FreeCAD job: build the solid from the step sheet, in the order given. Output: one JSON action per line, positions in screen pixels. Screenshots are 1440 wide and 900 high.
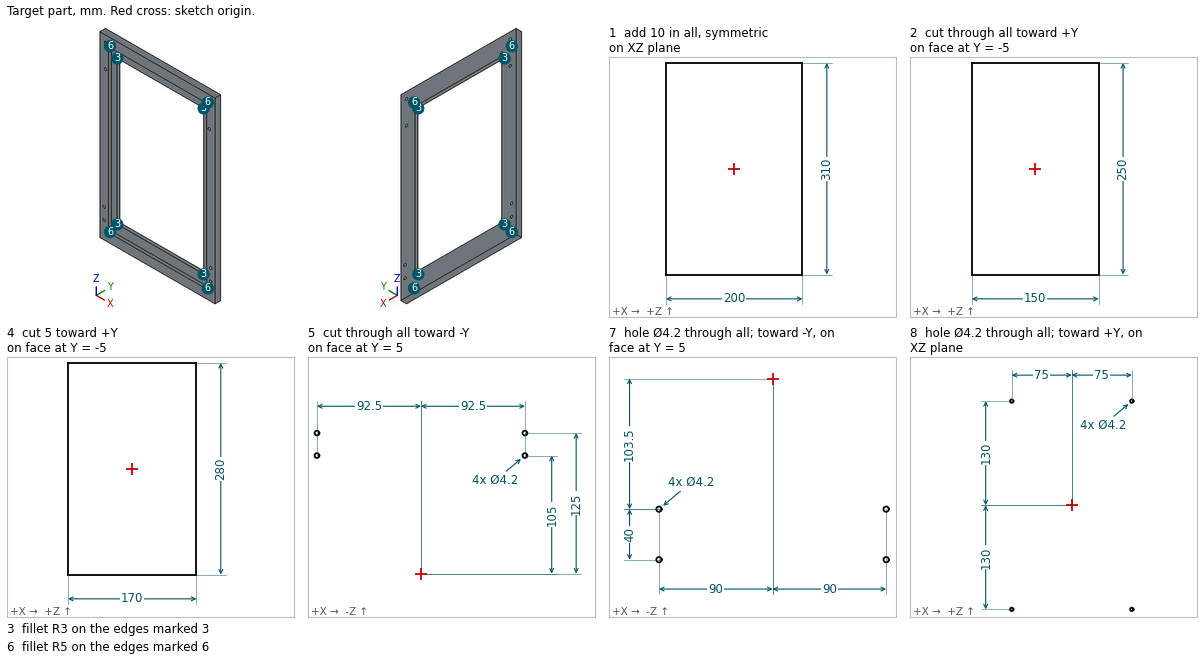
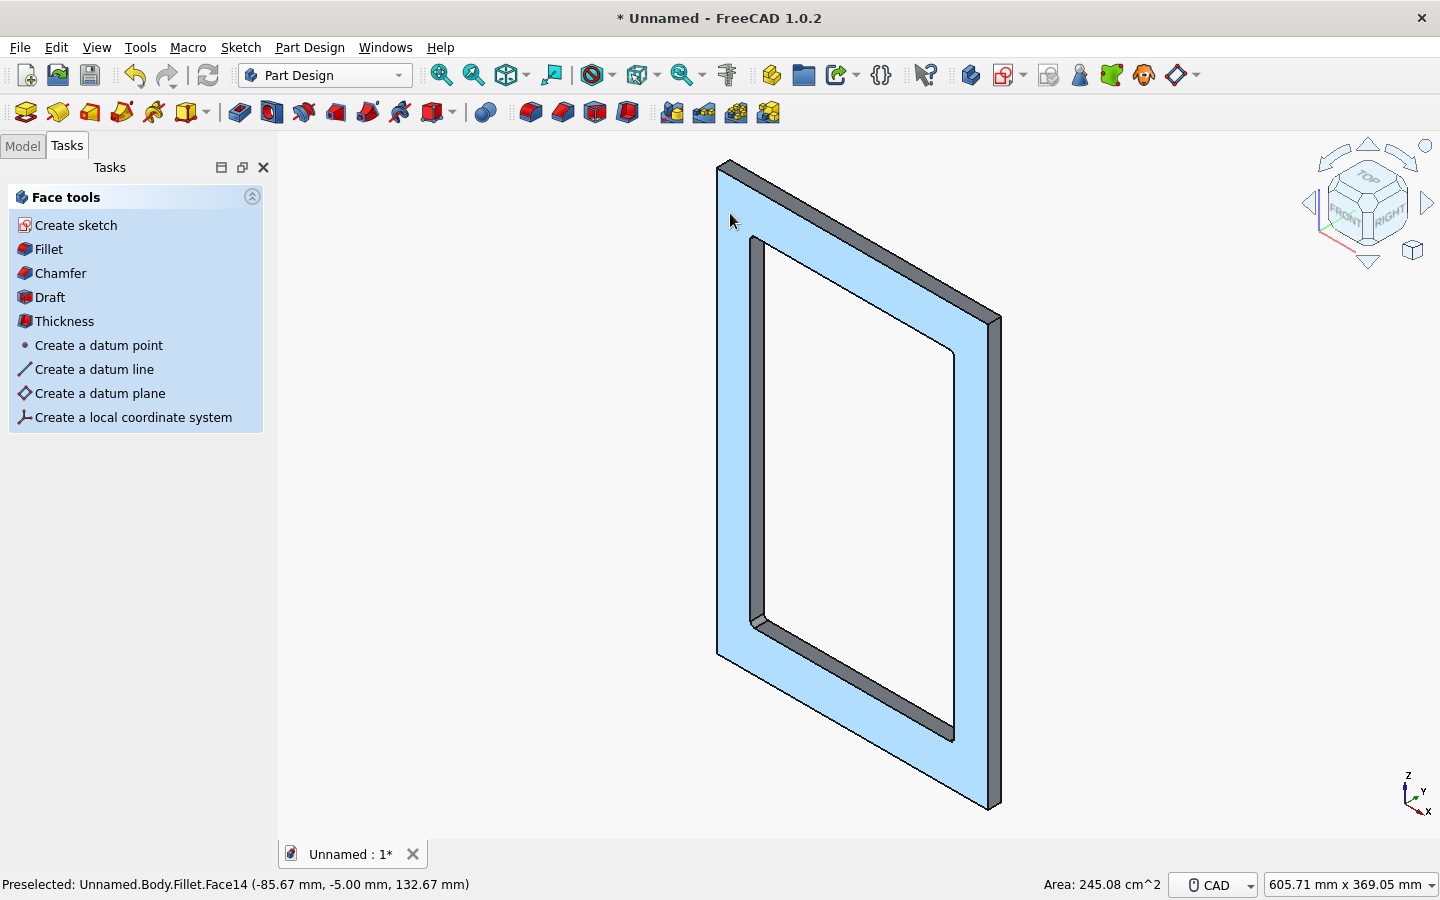
{"action": "left_click", "coordinate": [1004, 76]}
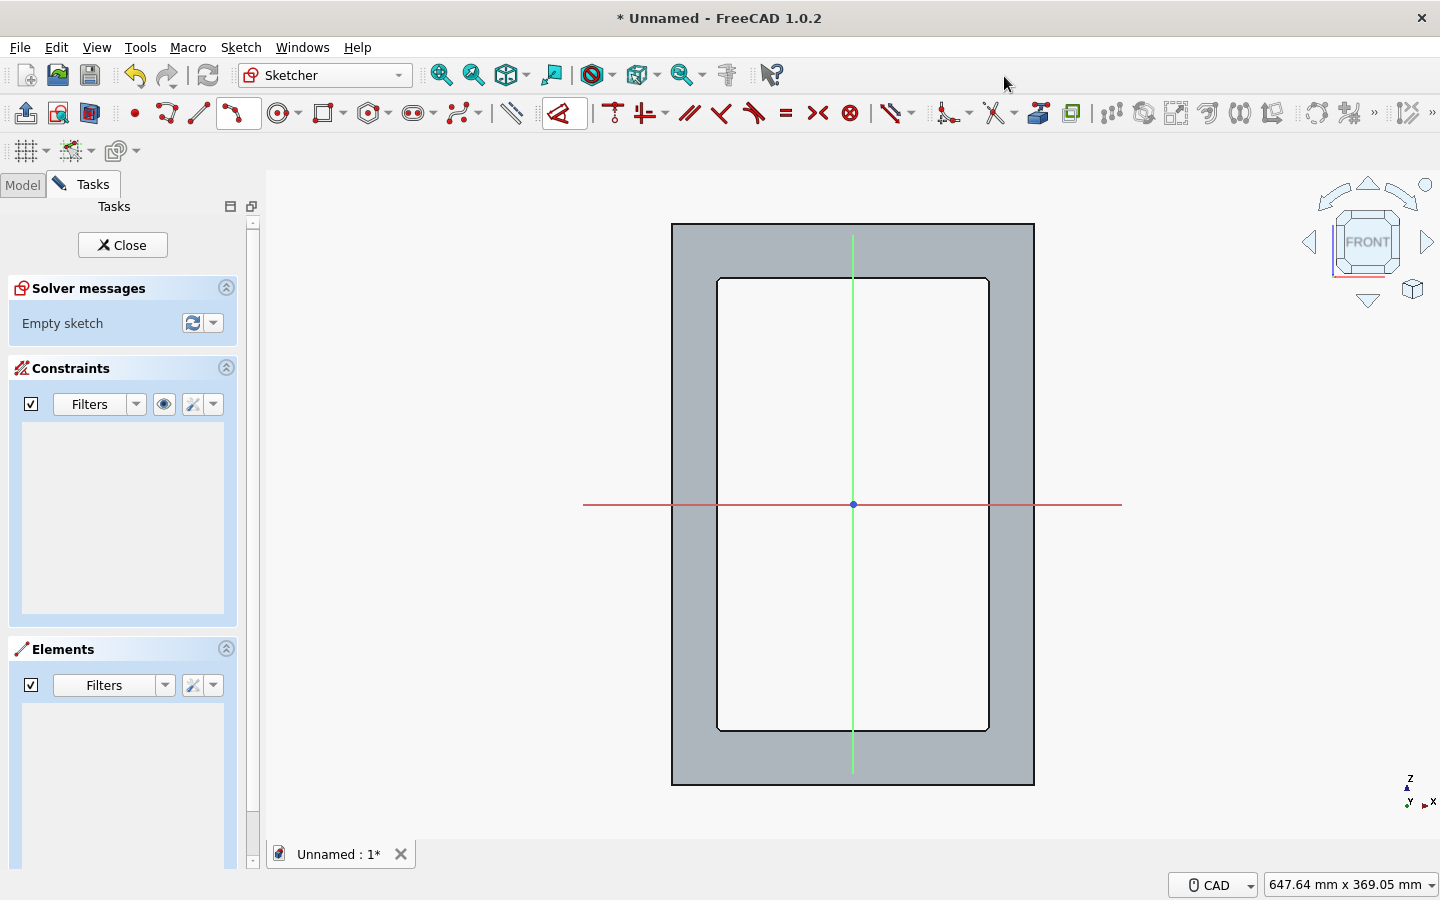
{"action": "key", "text": "g v"}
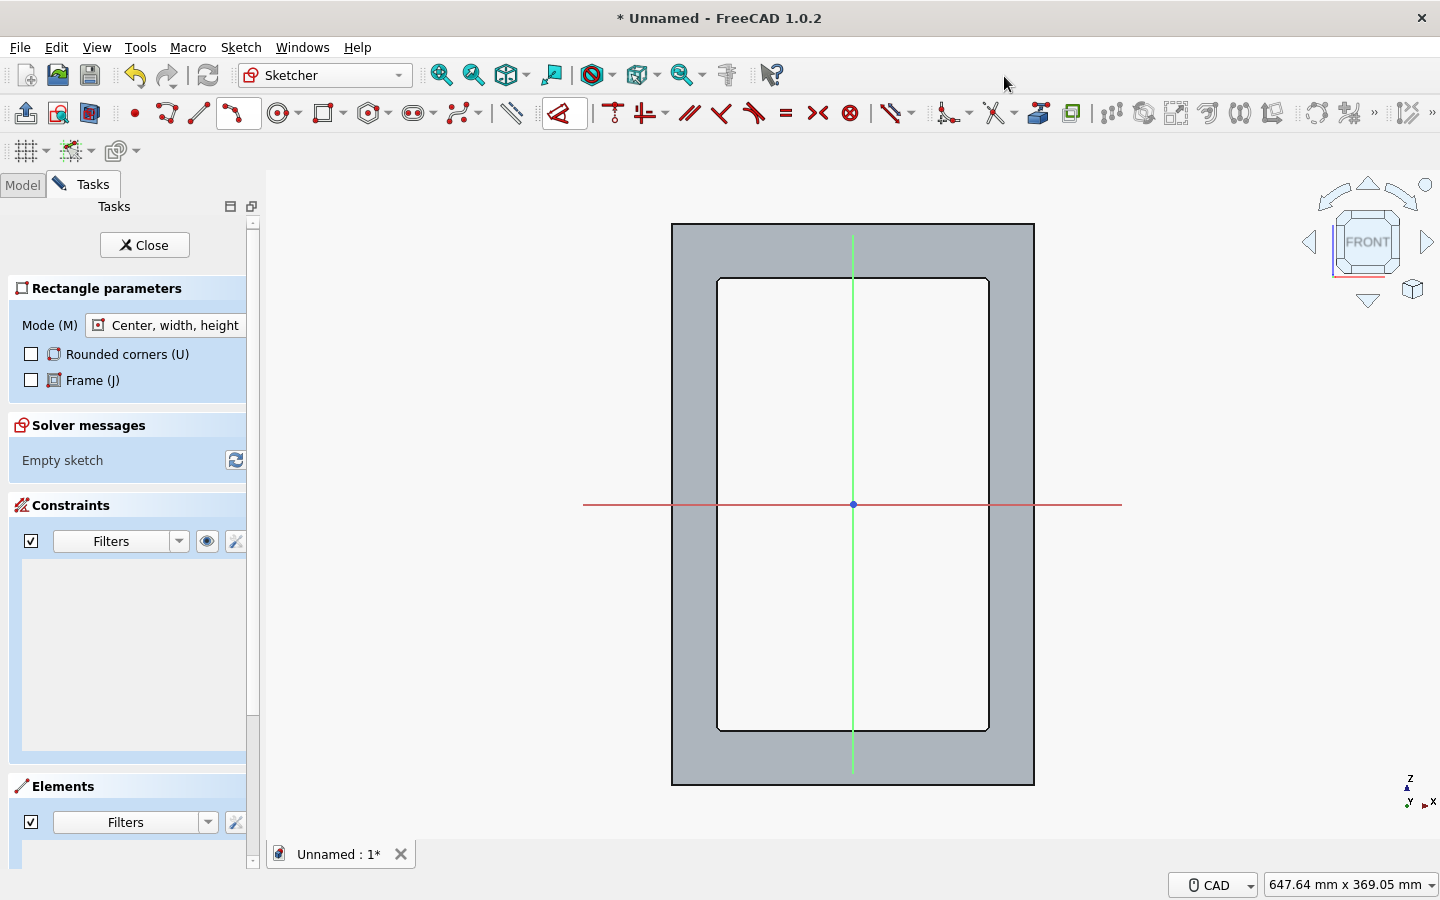
{"action": "left_click", "coordinate": [853, 504]}
{"action": "left_click", "coordinate": [1007, 251]}
{"action": "key", "text": "Escape"}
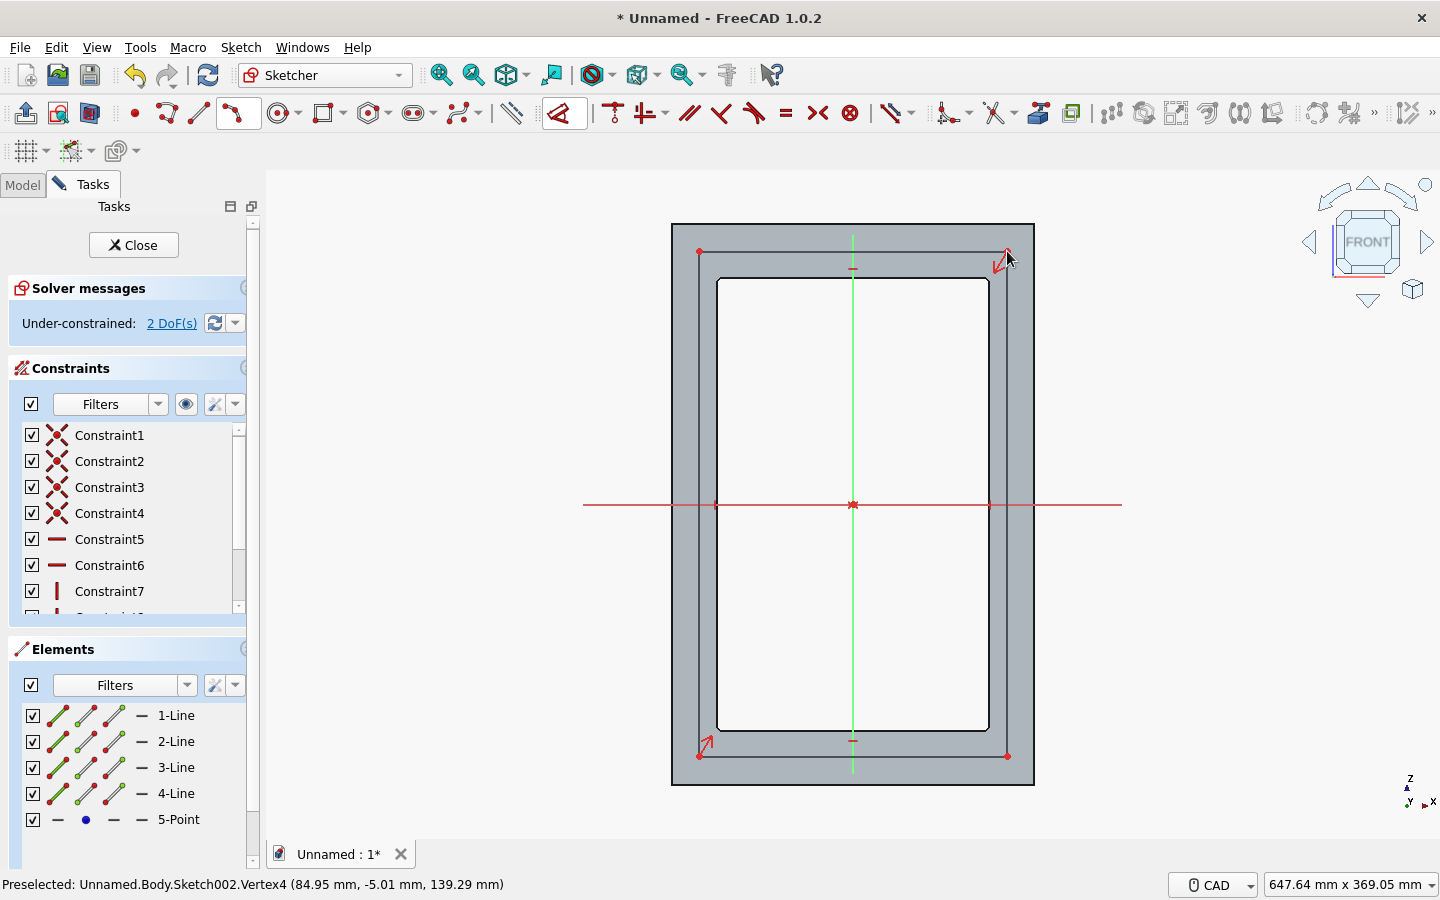
{"action": "left_click", "coordinate": [791, 757]}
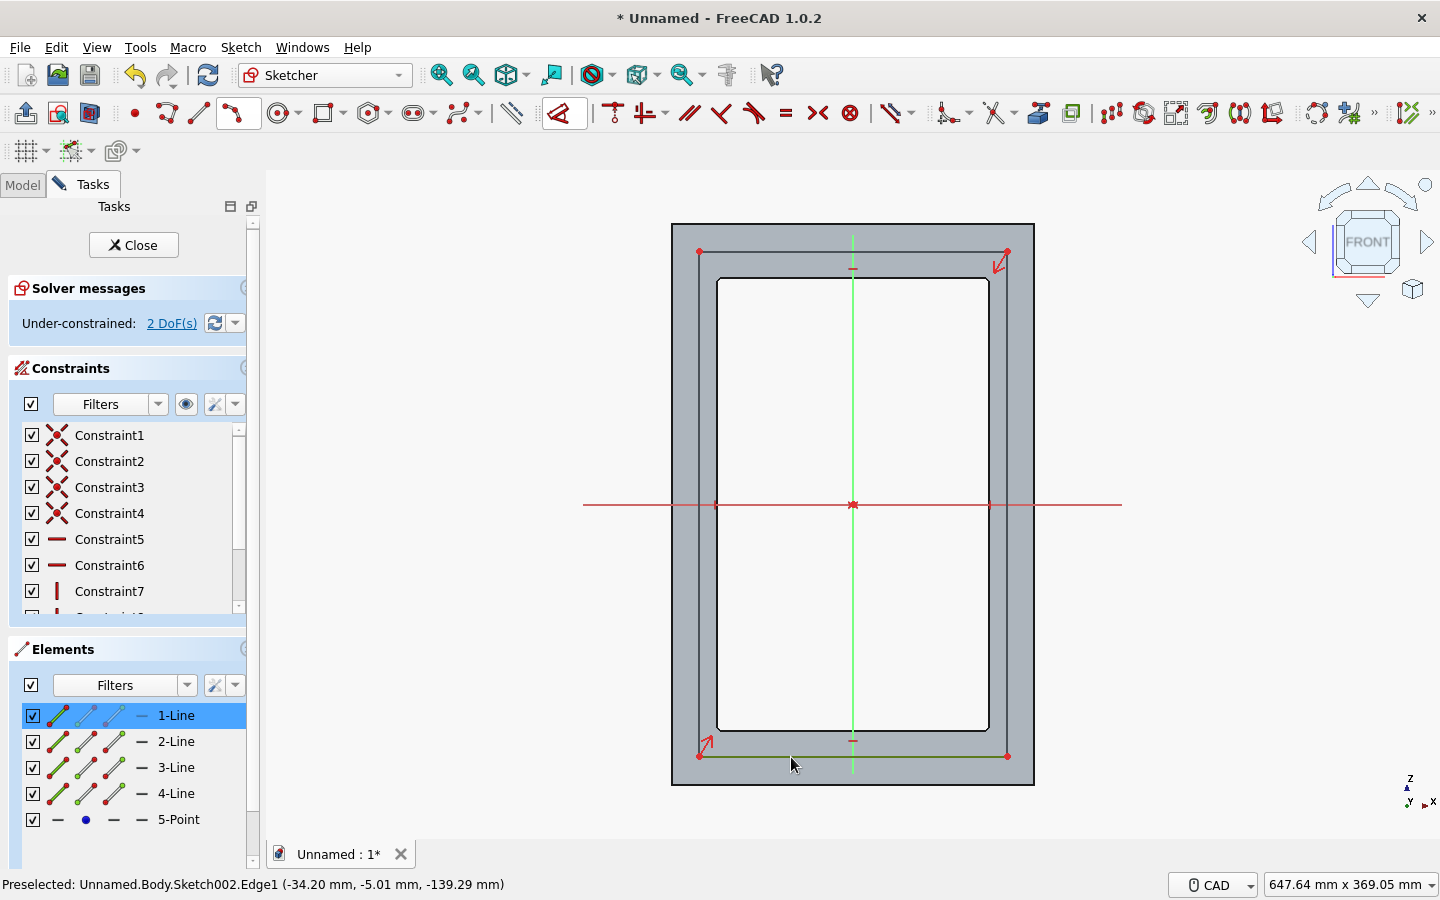
{"action": "key", "text": "l"}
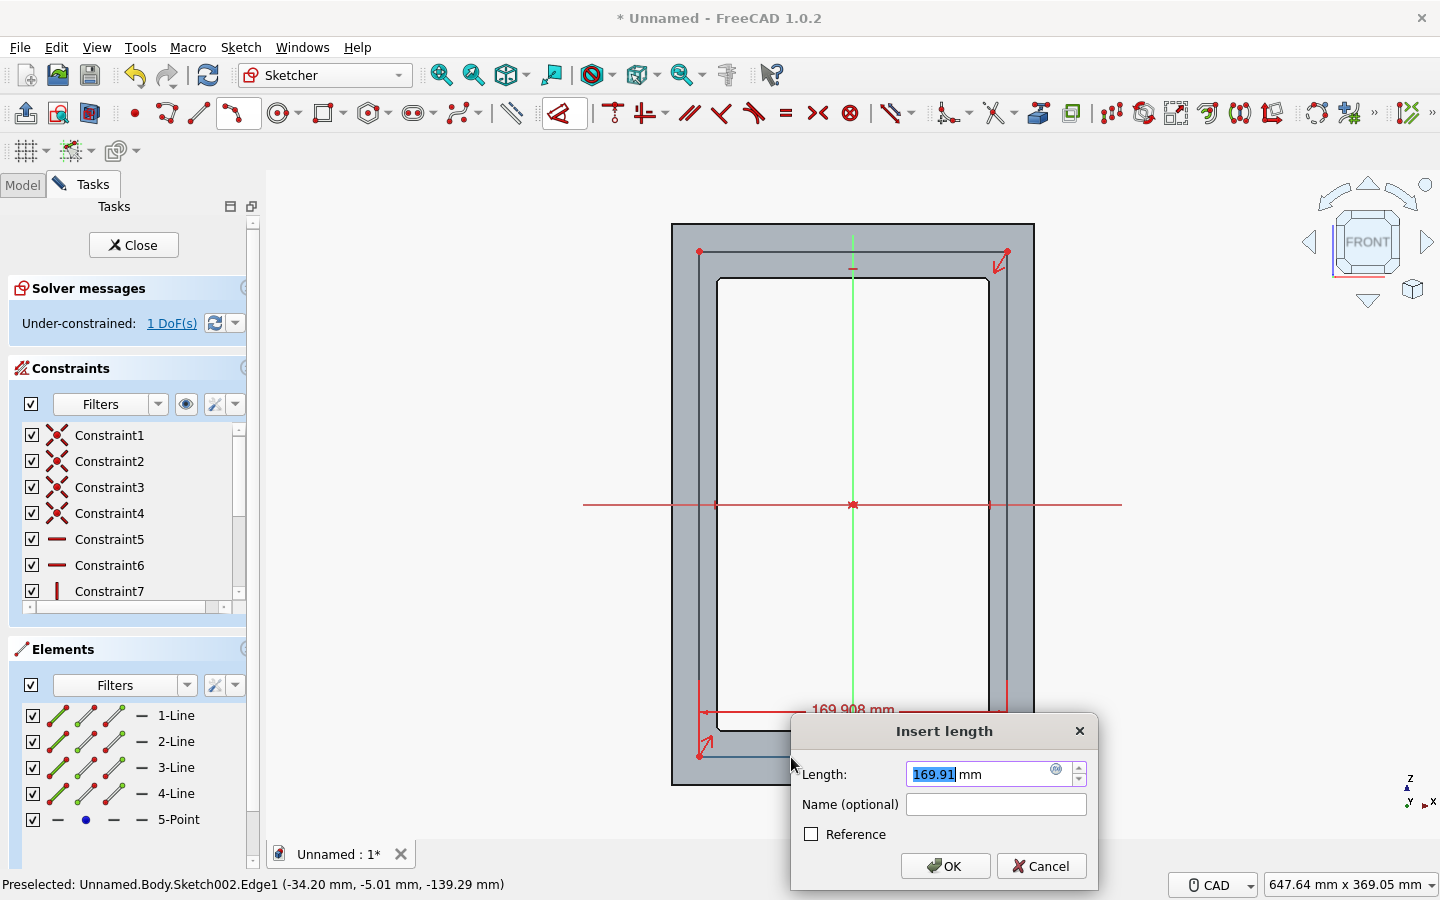
{"action": "type", "text": "170"}
{"action": "key", "text": "Return"}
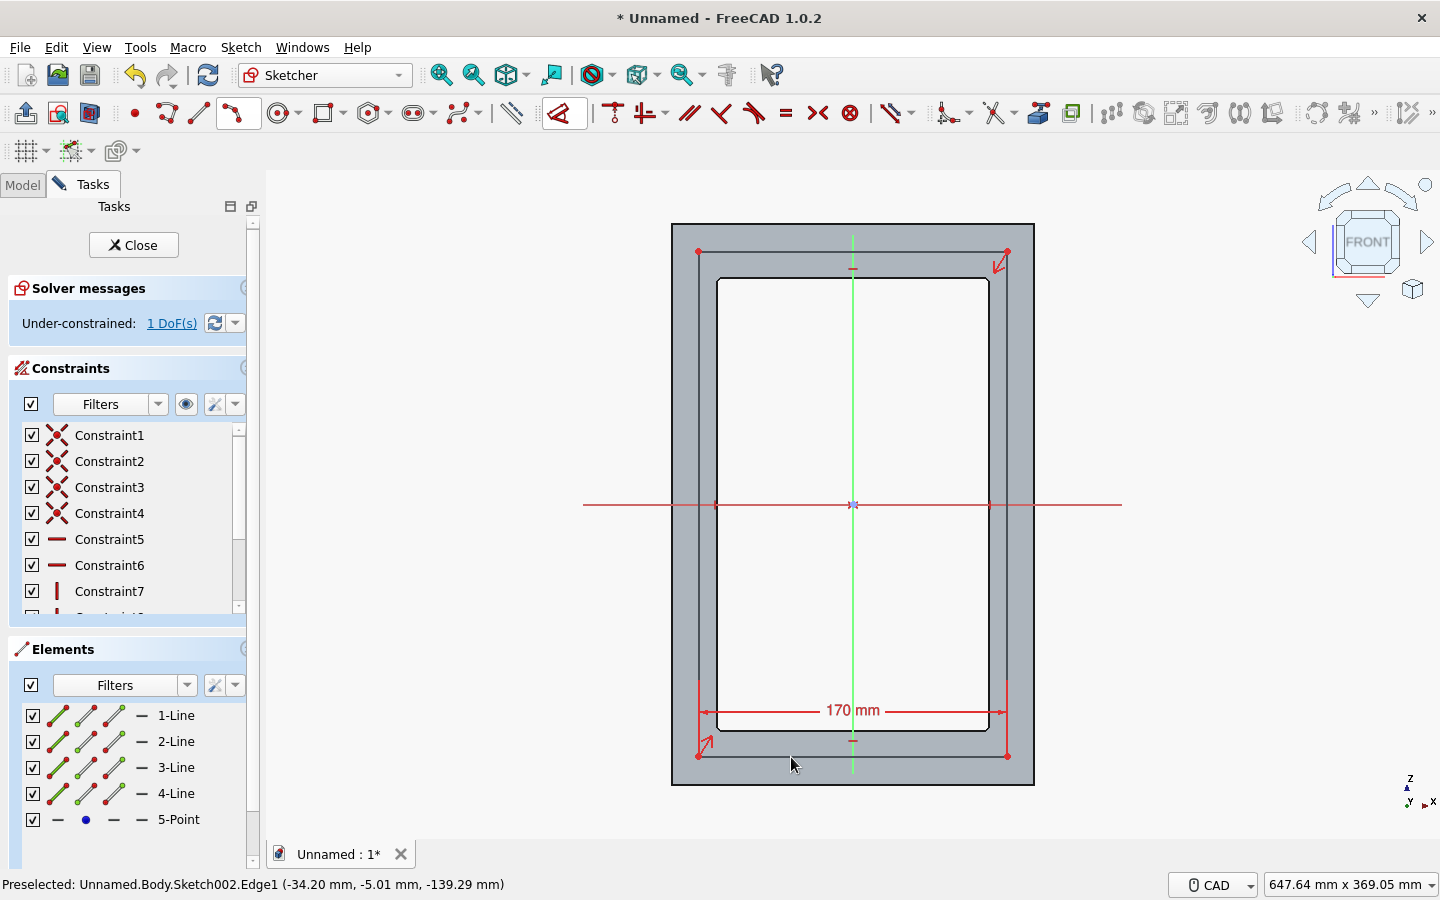
{"action": "left_click", "coordinate": [1007, 605]}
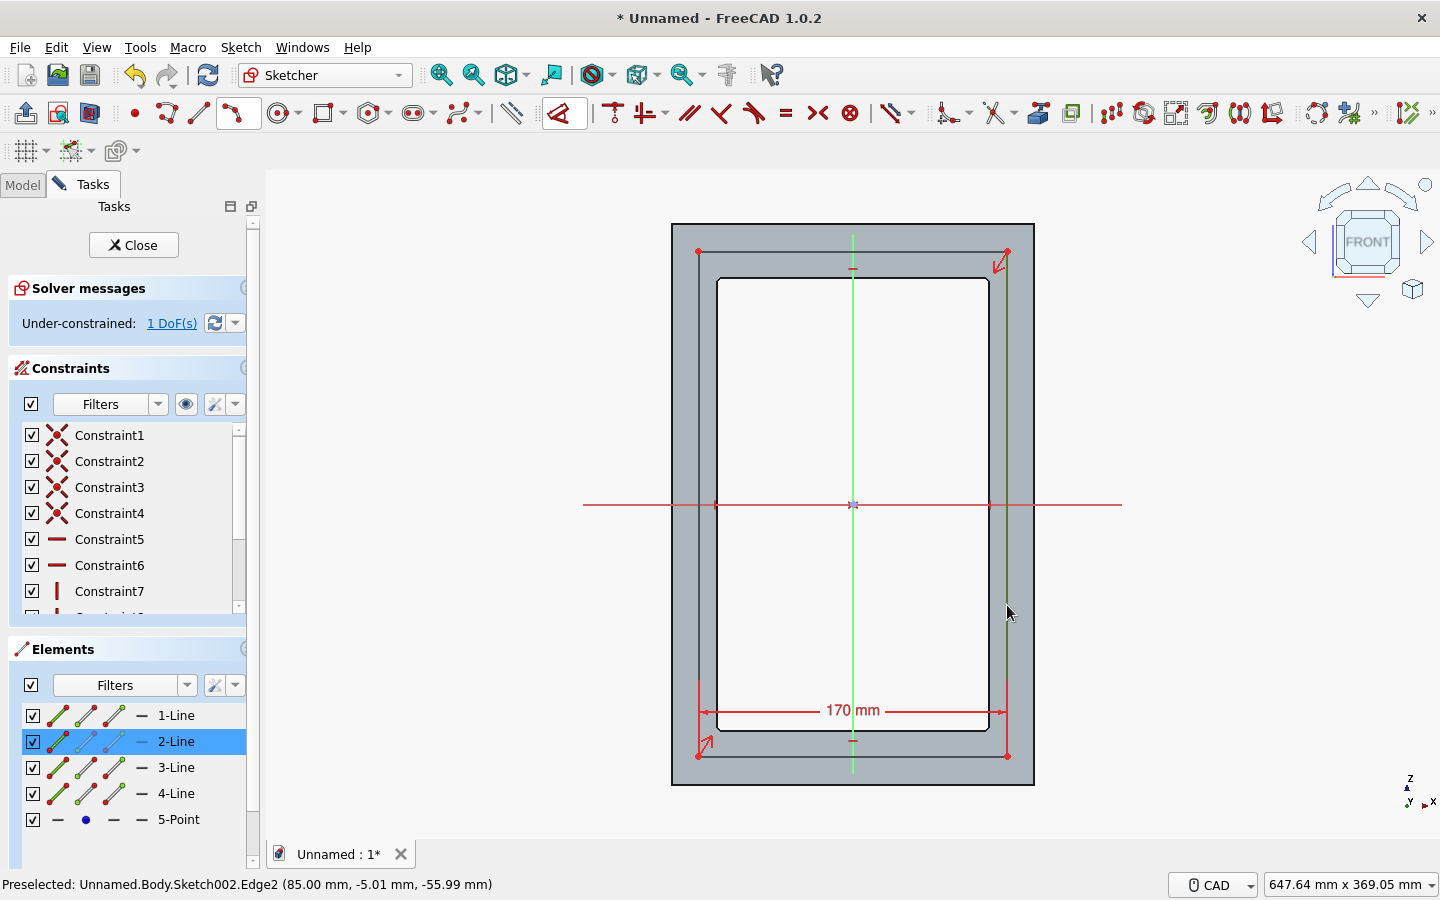
{"action": "key", "text": "i"}